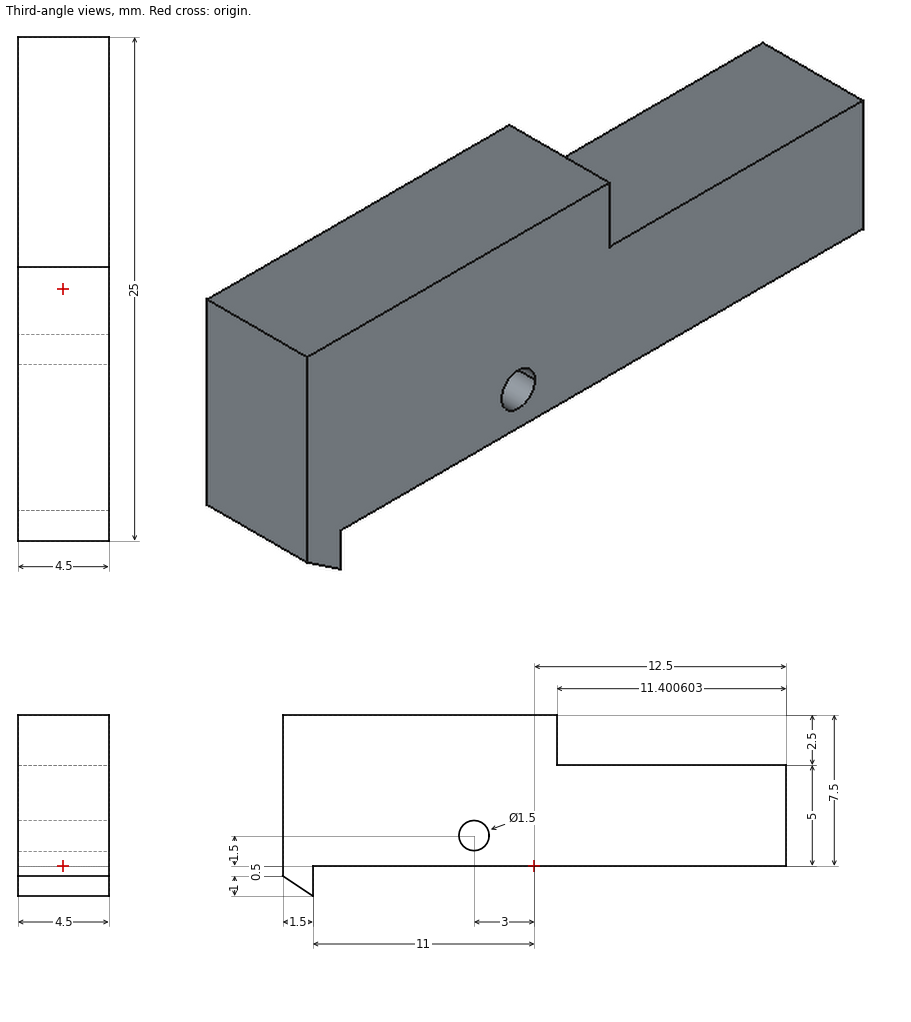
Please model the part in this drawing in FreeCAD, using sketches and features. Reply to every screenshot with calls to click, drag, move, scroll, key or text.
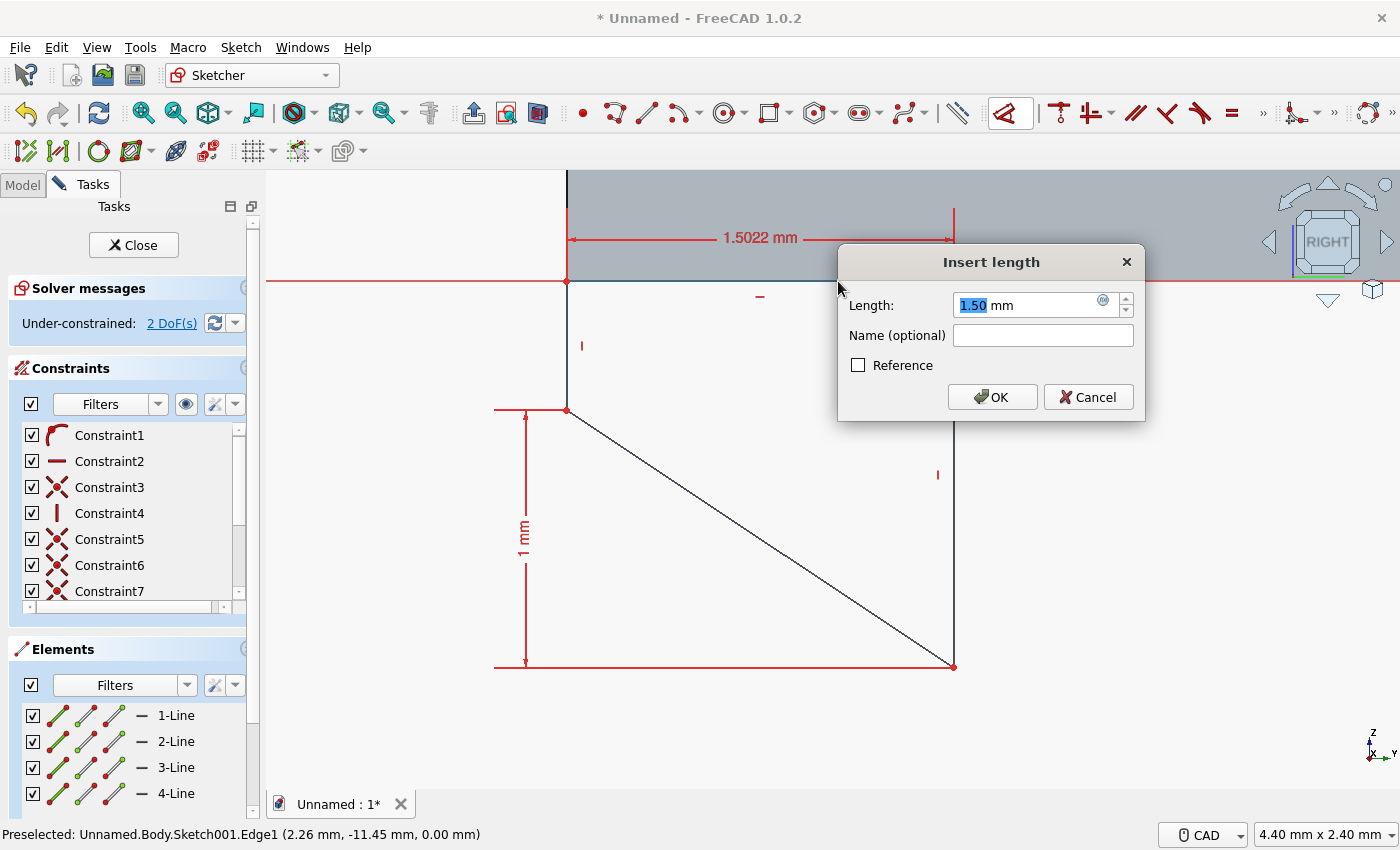
text(1.5)
key(Return)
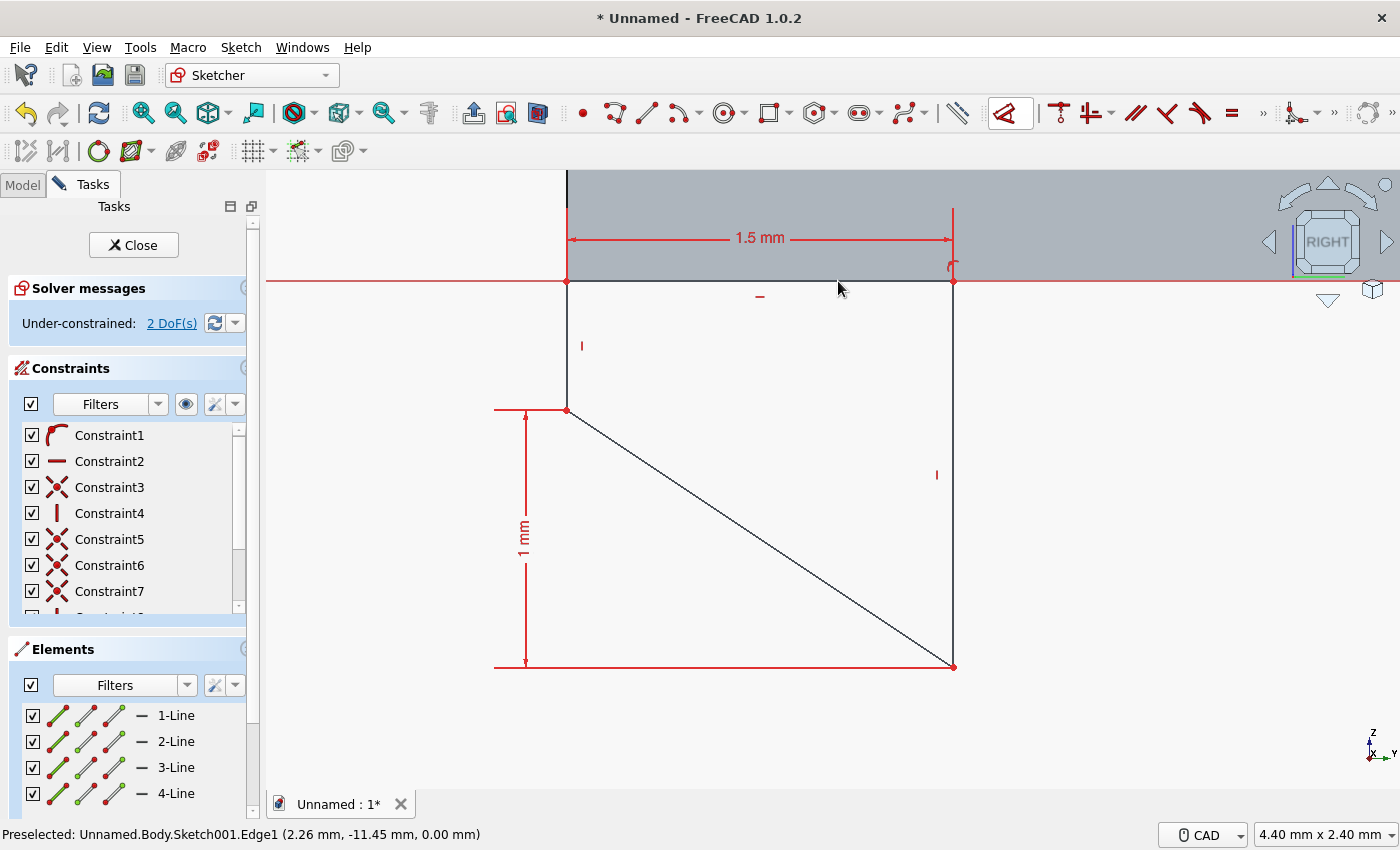
click(567, 320)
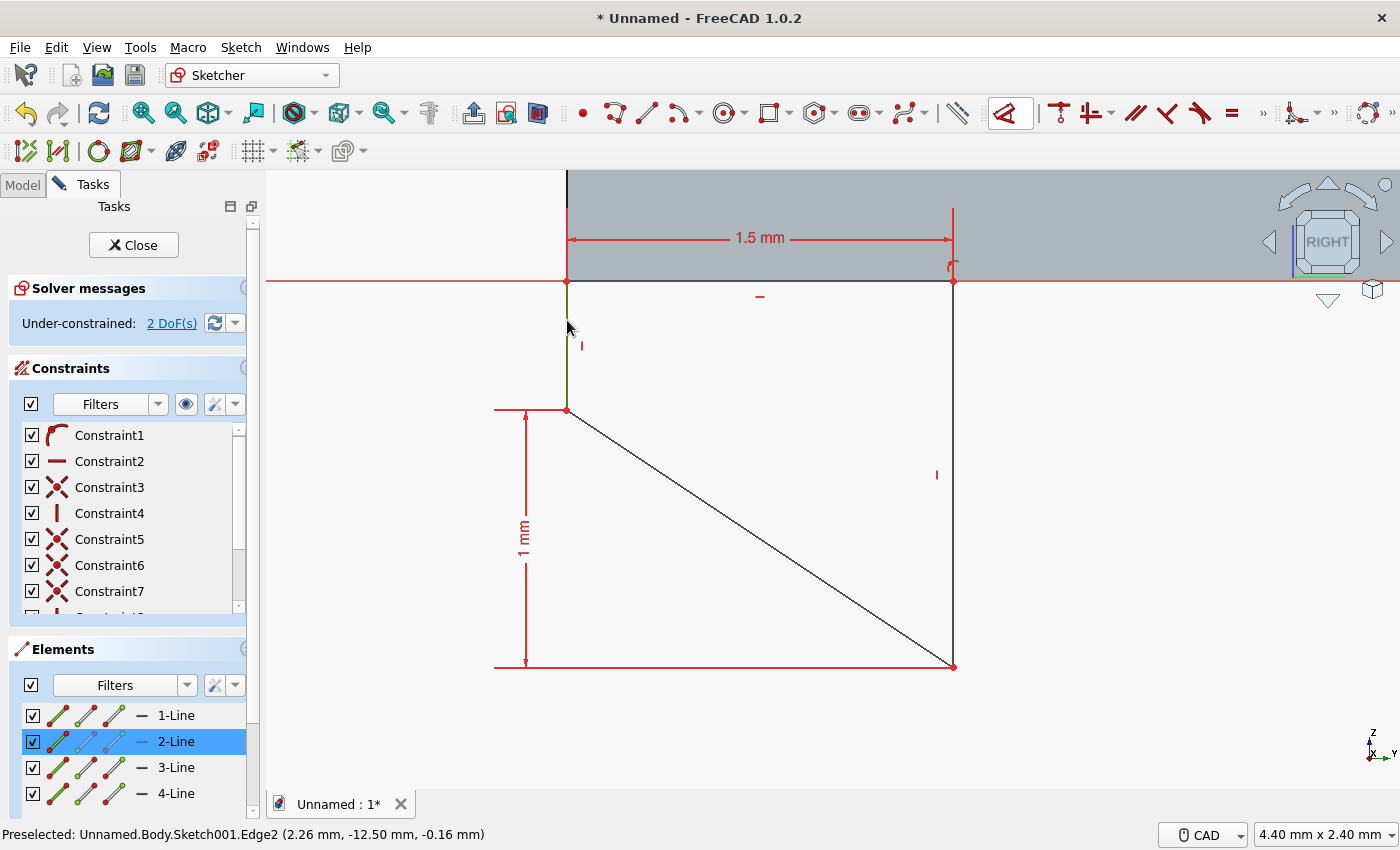
key(i)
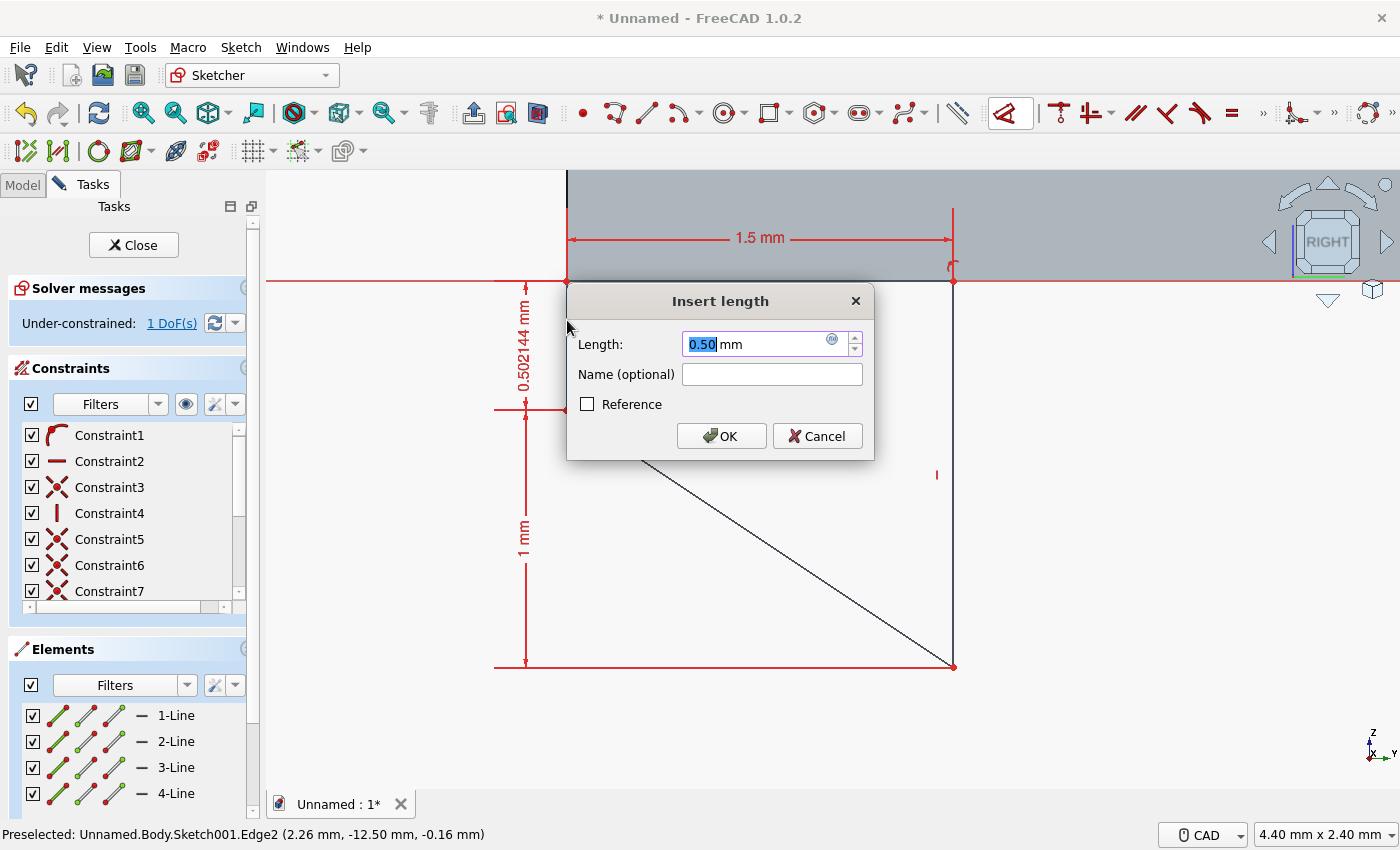
text(0.5)
key(Return)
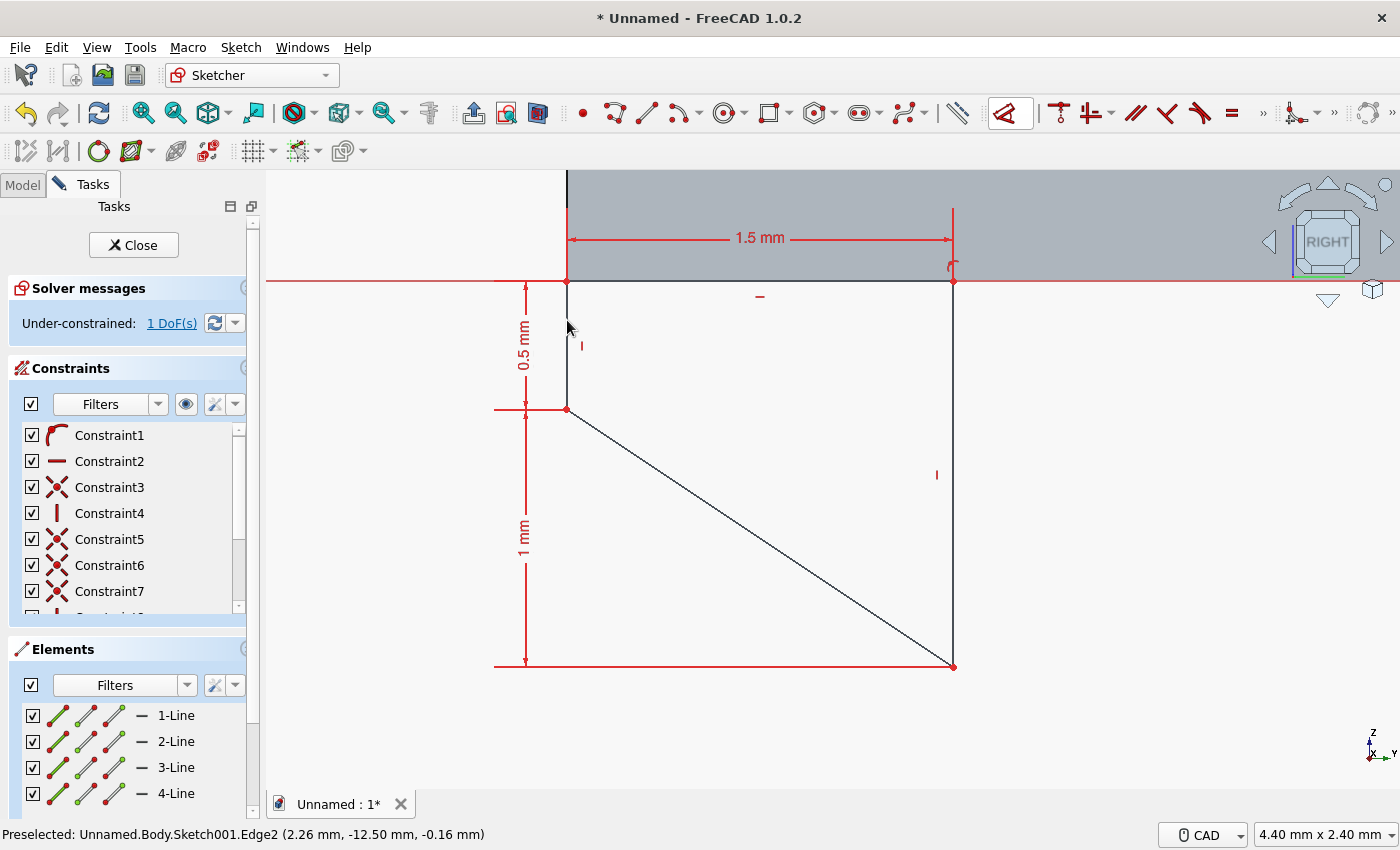
click(953, 281)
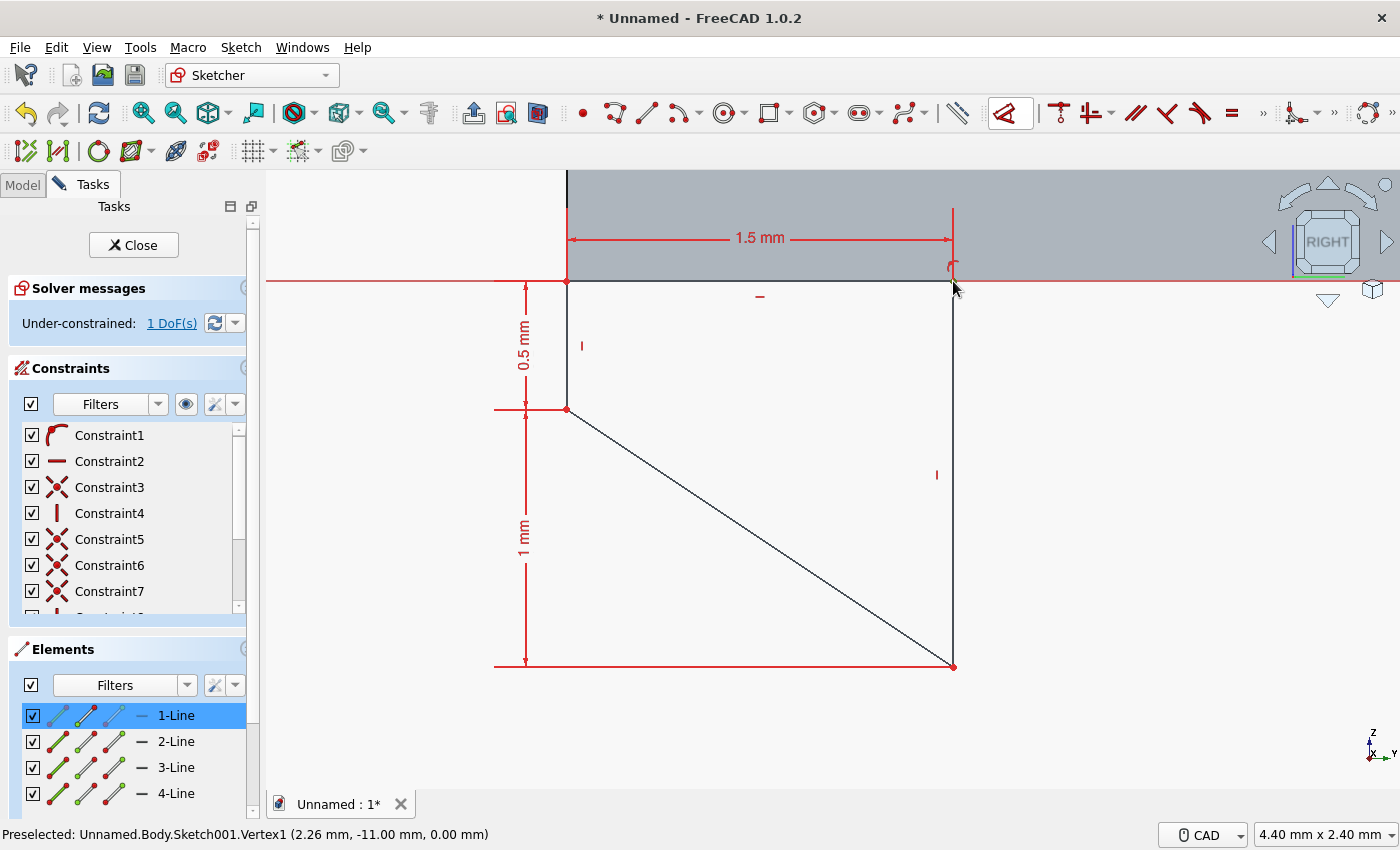
click(1028, 114)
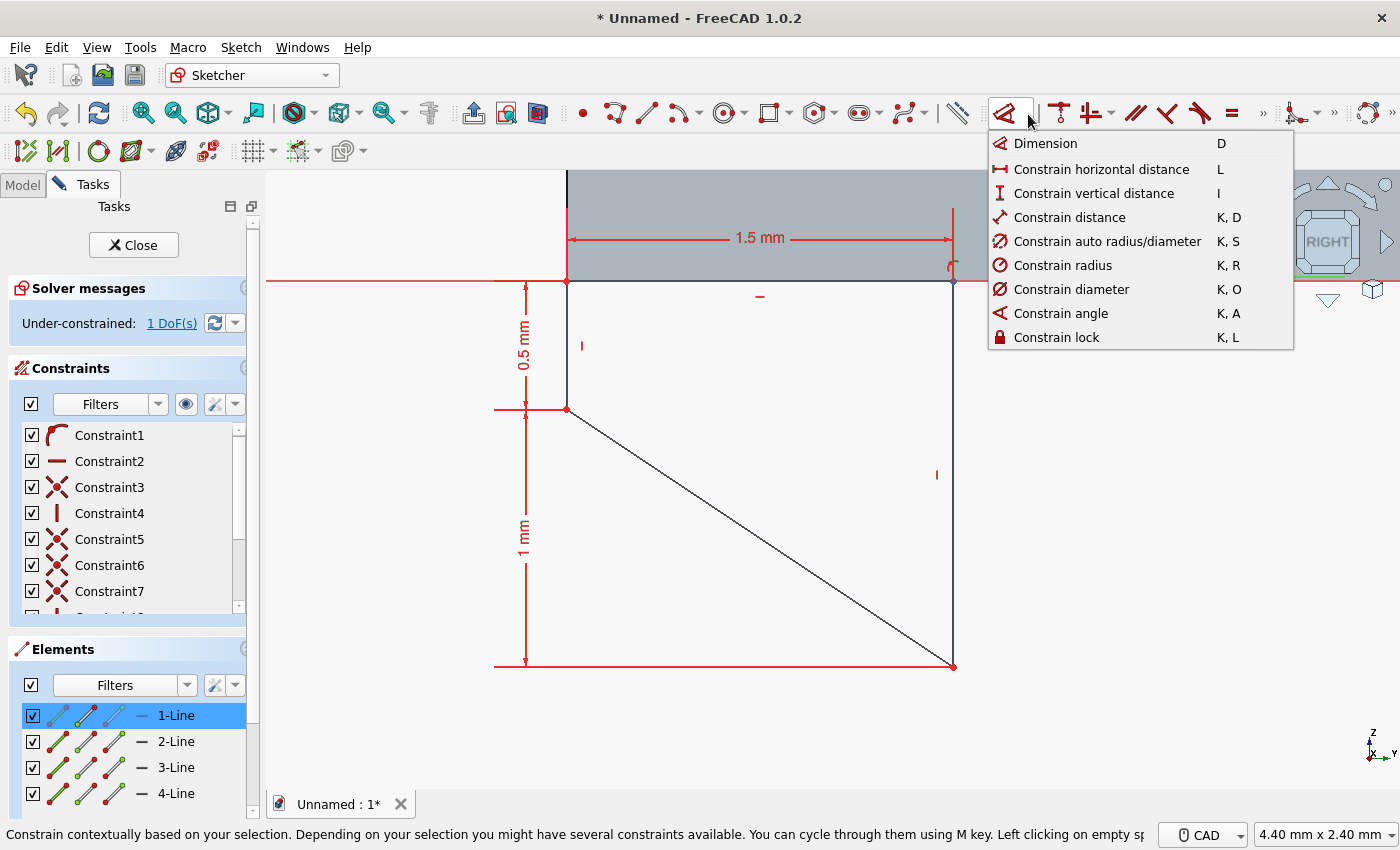
click(1141, 169)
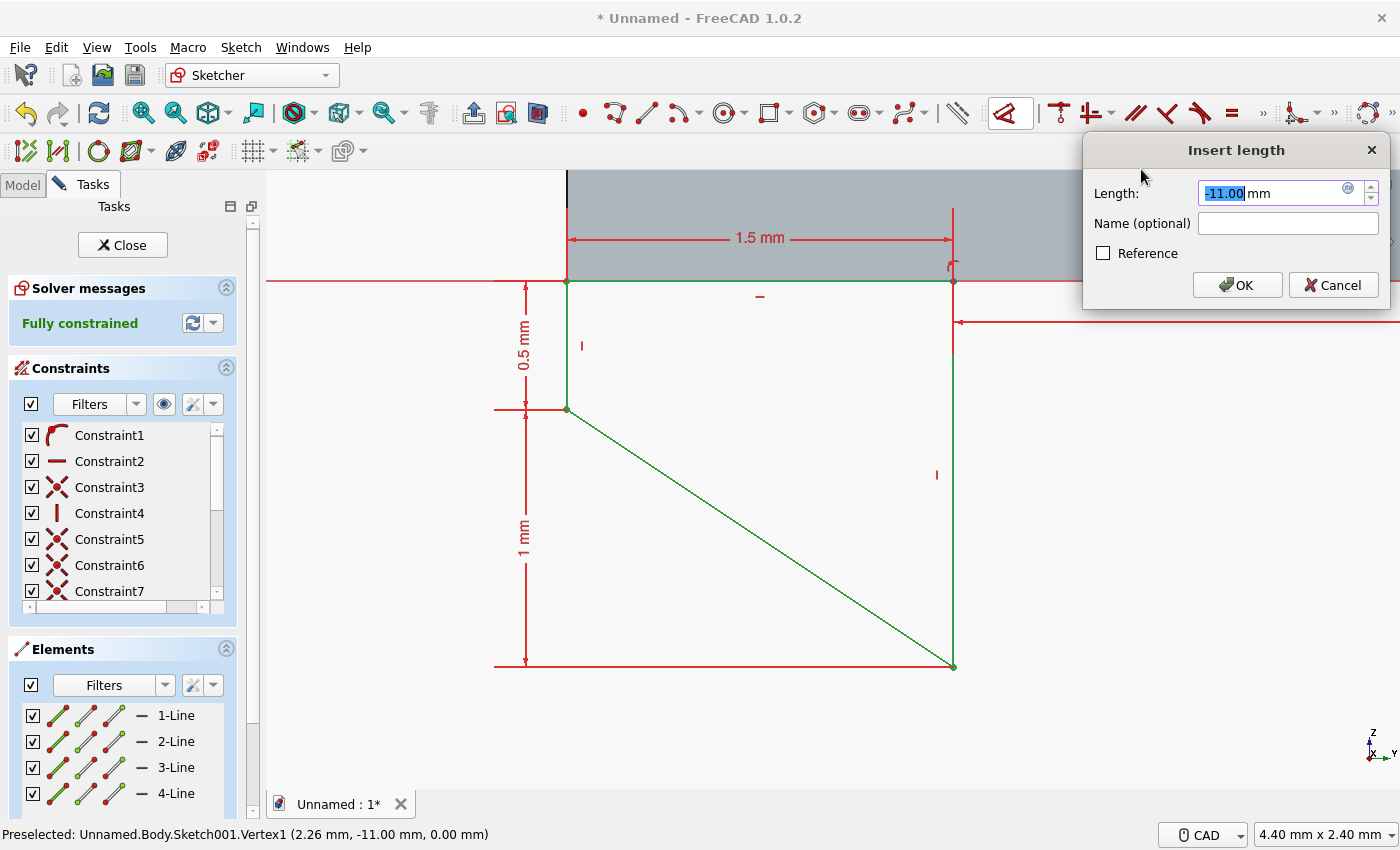
text(-11)
key(Return)